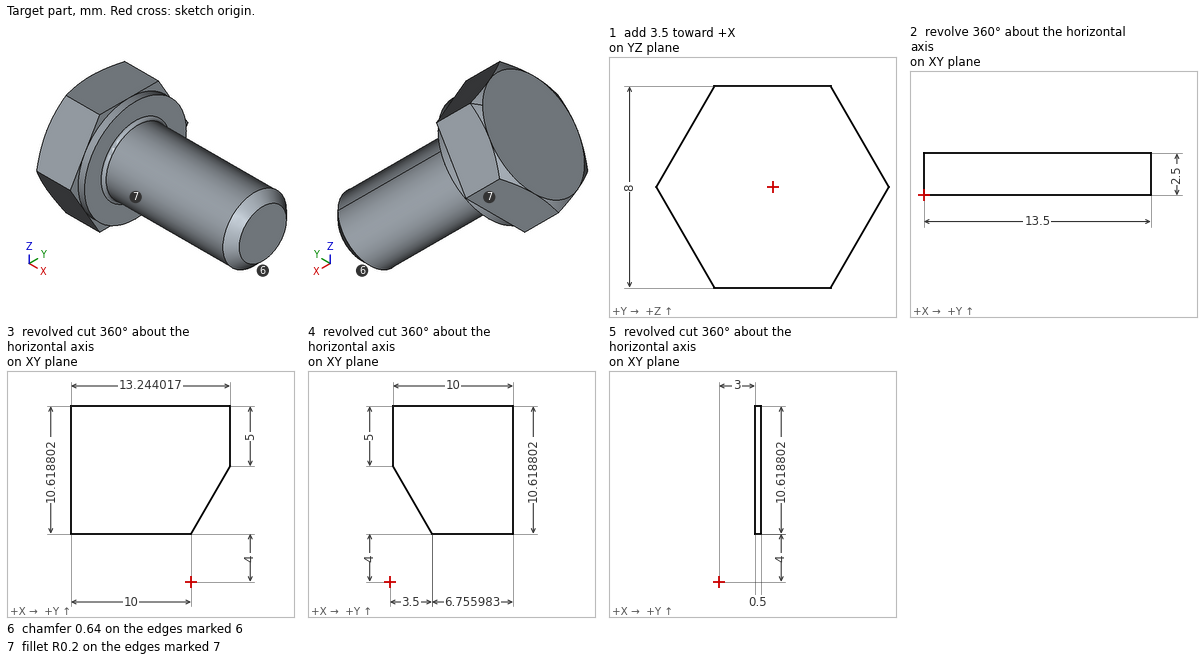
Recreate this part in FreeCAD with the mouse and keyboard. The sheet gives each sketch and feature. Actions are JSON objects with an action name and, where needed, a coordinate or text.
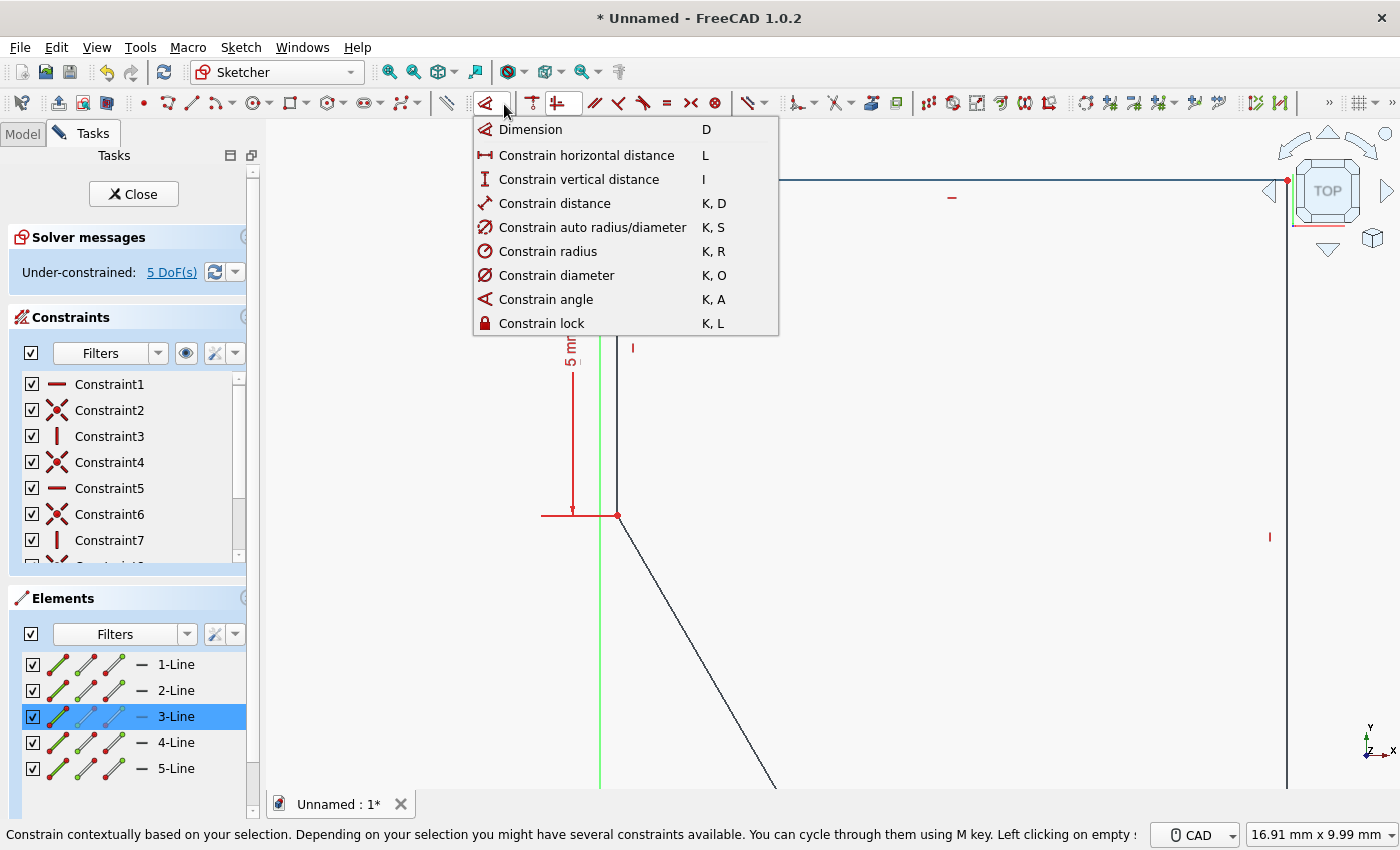
{"action": "left_click", "coordinate": [626, 155]}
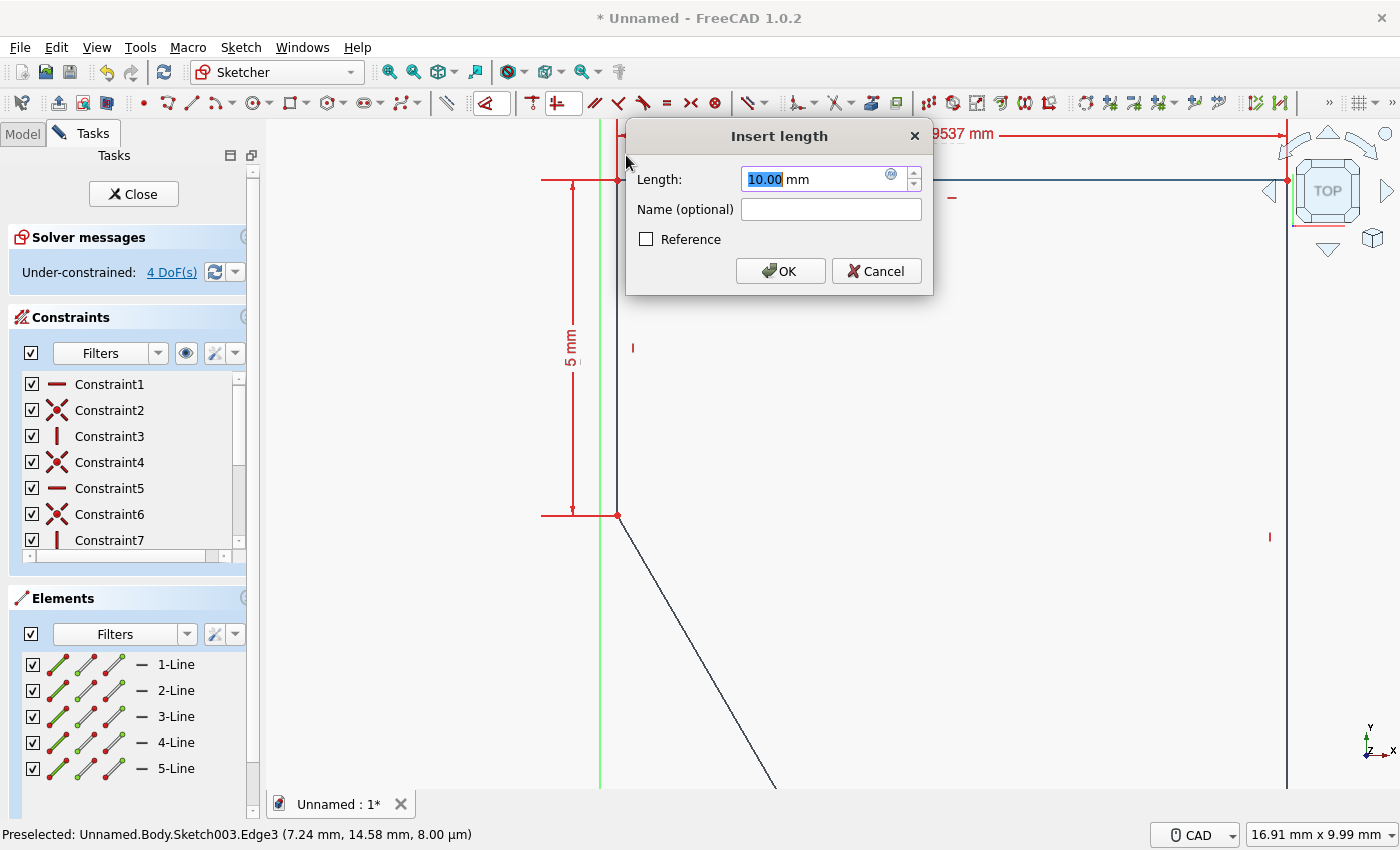
{"action": "type", "text": "10"}
{"action": "key", "text": "Return"}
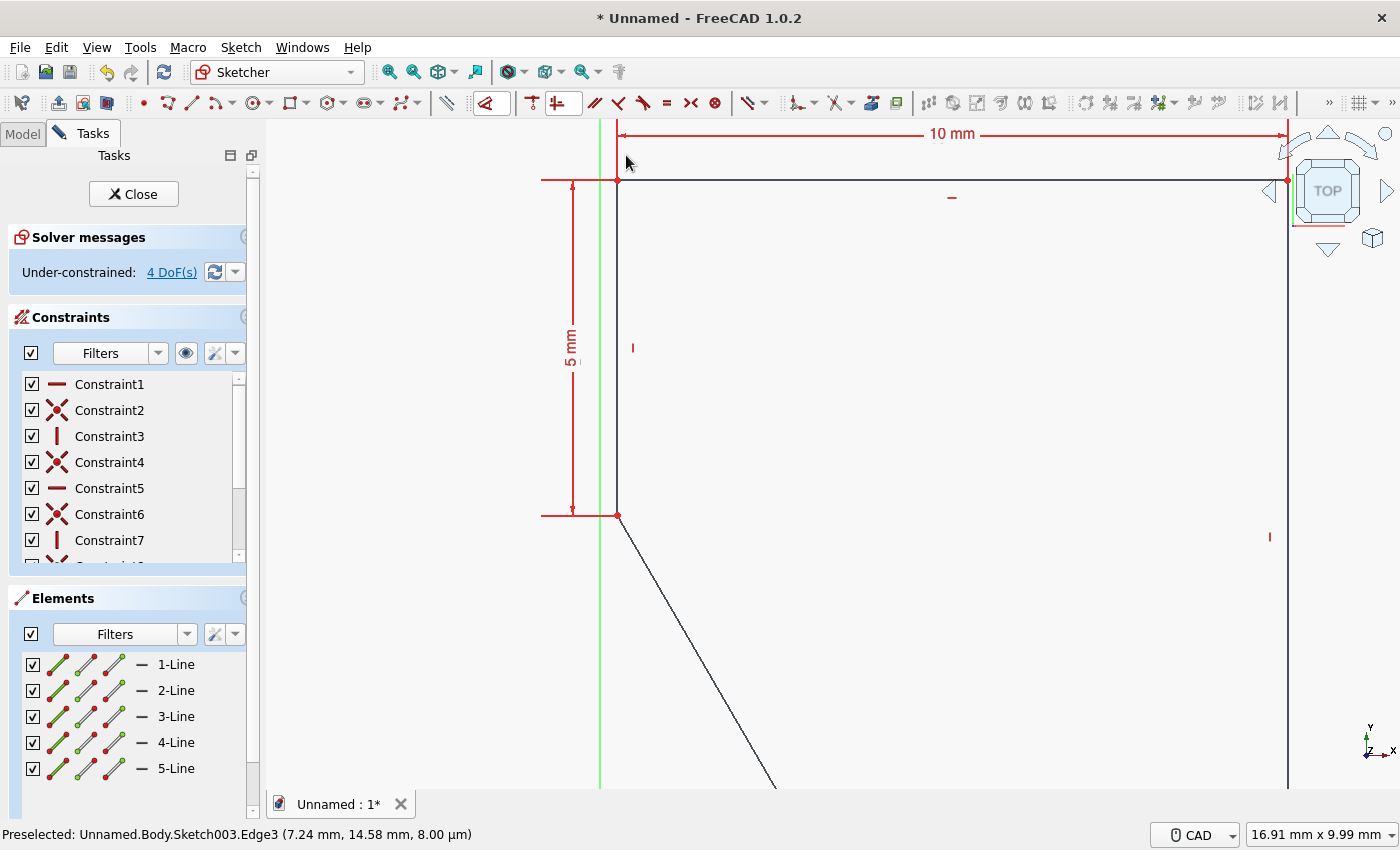
{"action": "scroll", "coordinate": [618, 280], "scroll_direction": "down", "scroll_amount": 4}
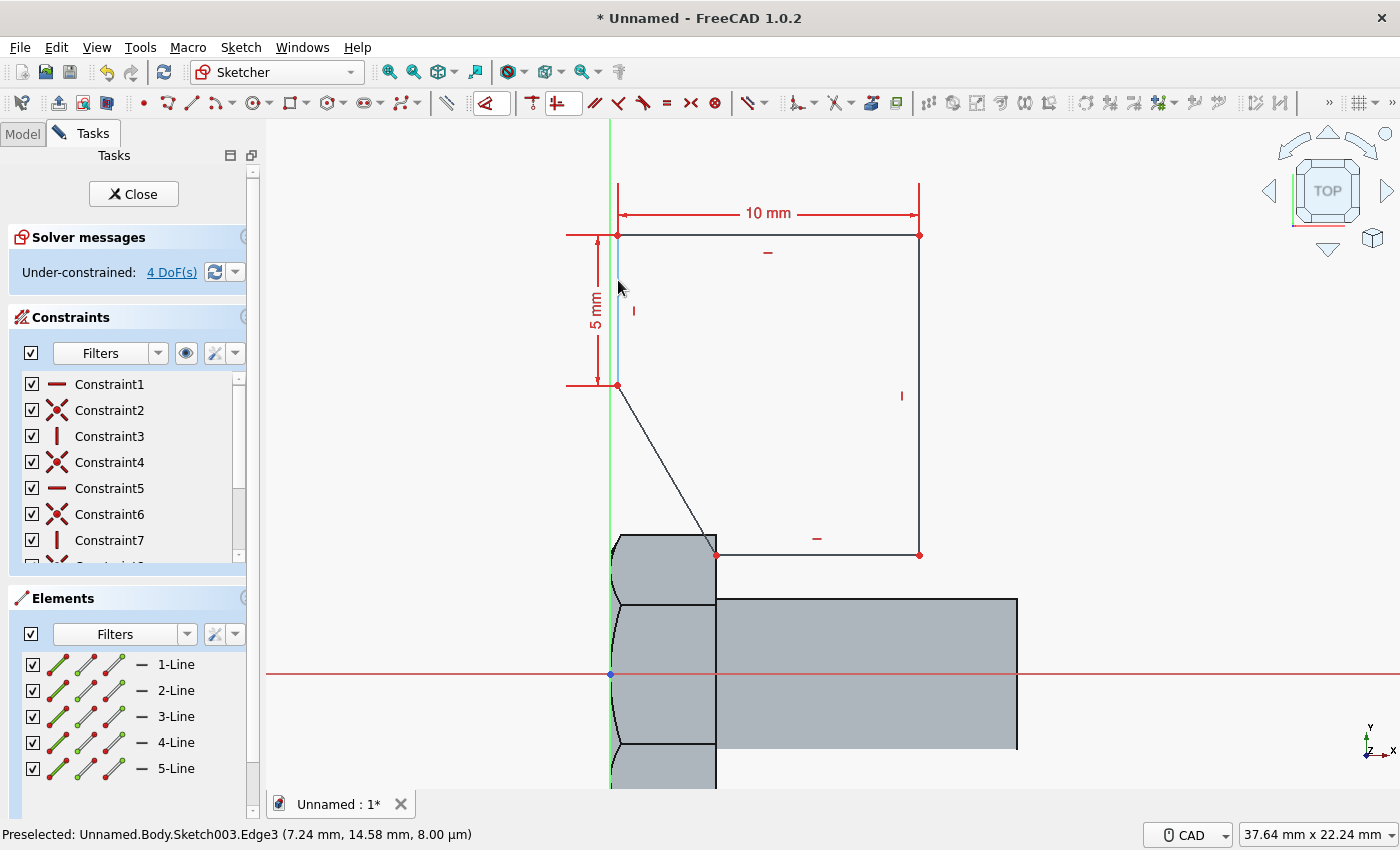
{"action": "left_click", "coordinate": [716, 555]}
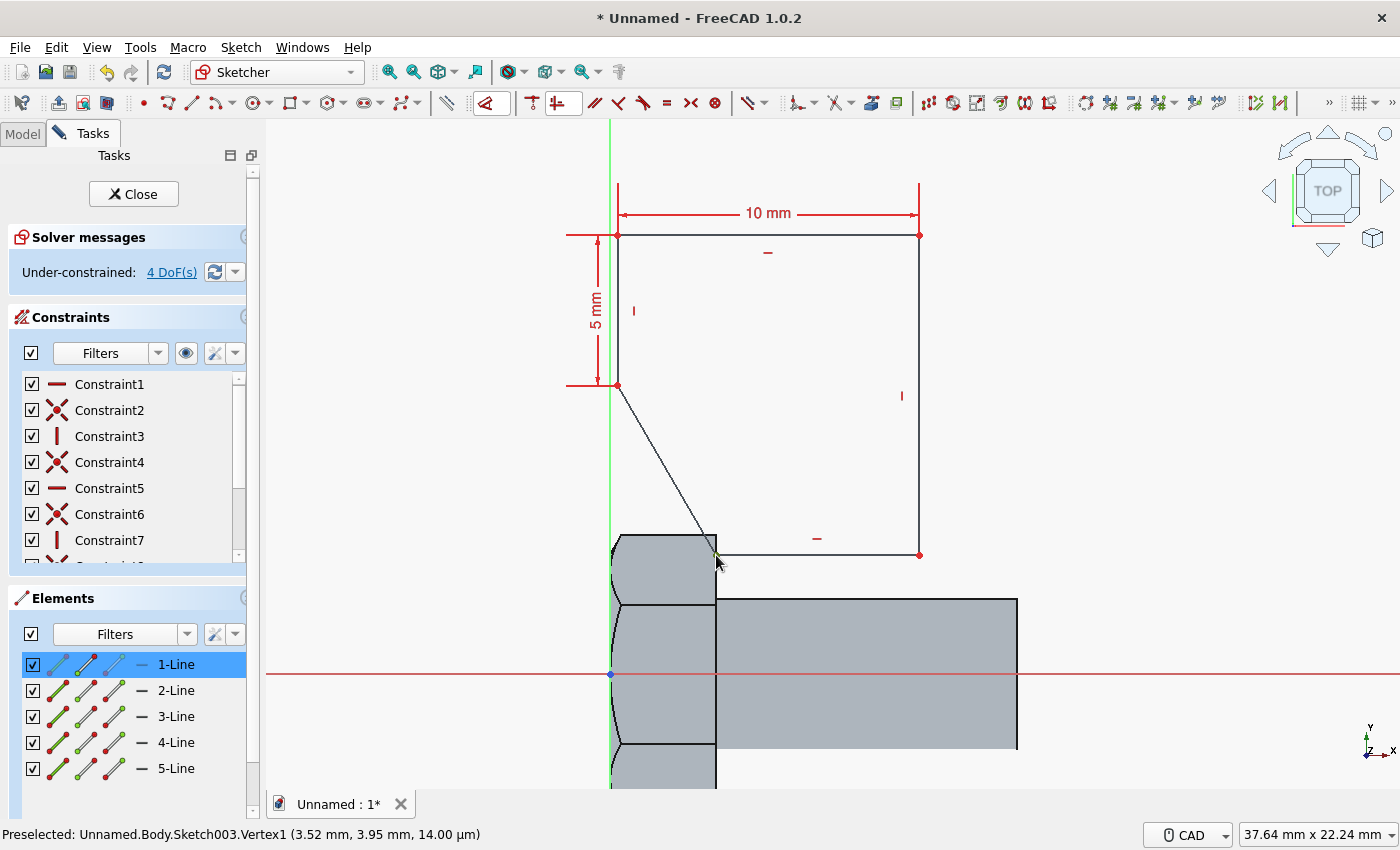
{"action": "key", "text": "i"}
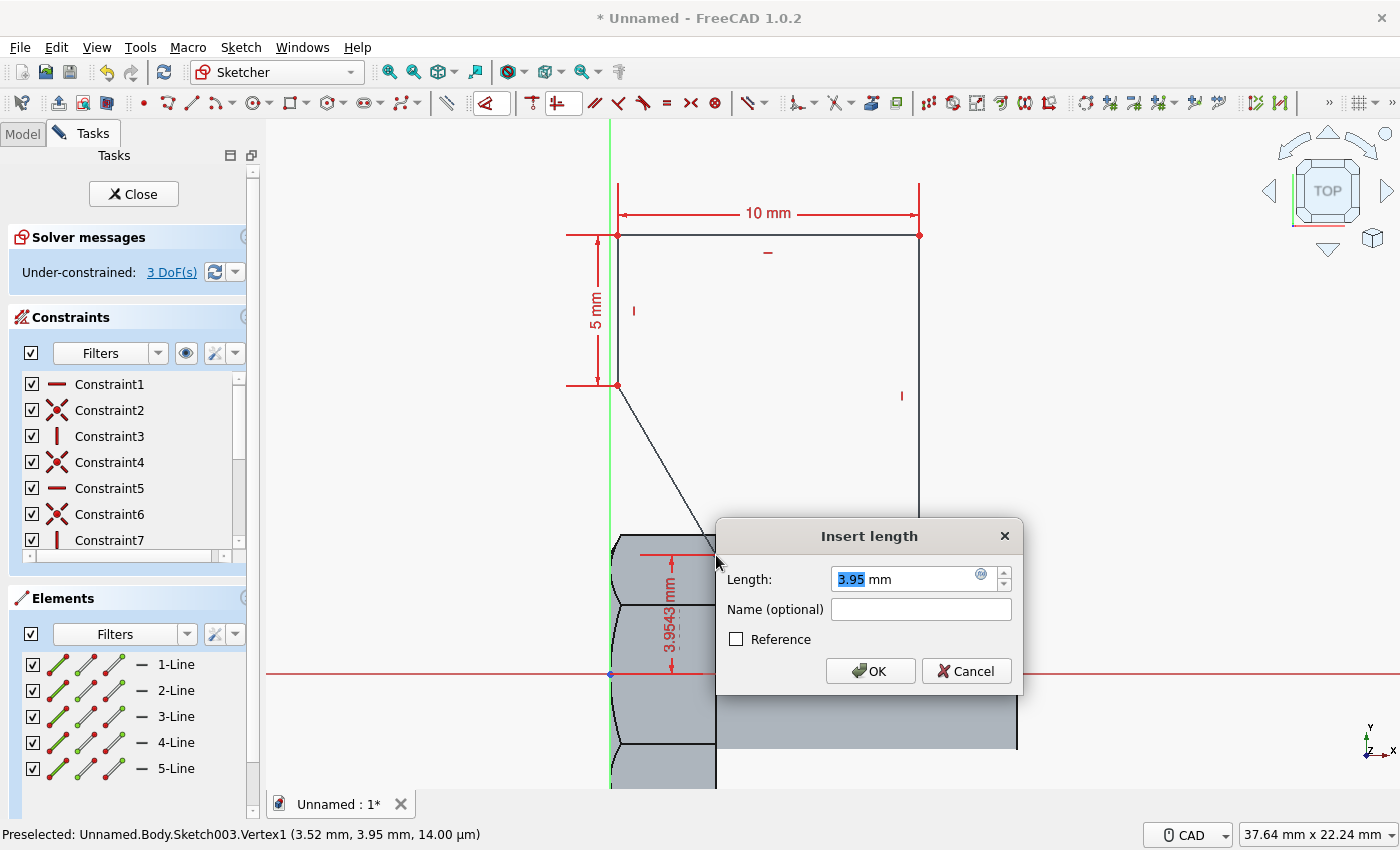
{"action": "type", "text": "4"}
{"action": "key", "text": "Return"}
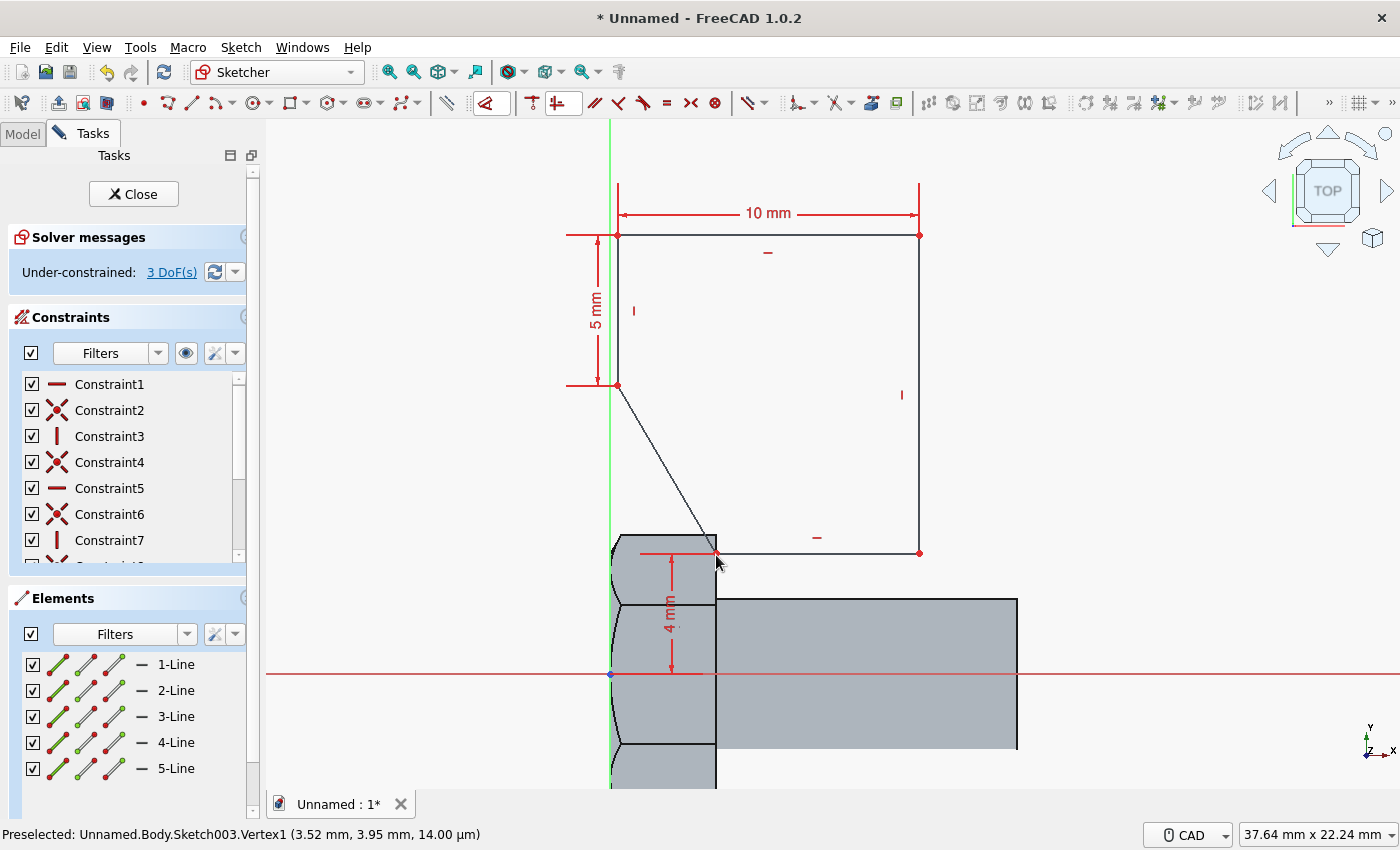
{"action": "left_click", "coordinate": [716, 554]}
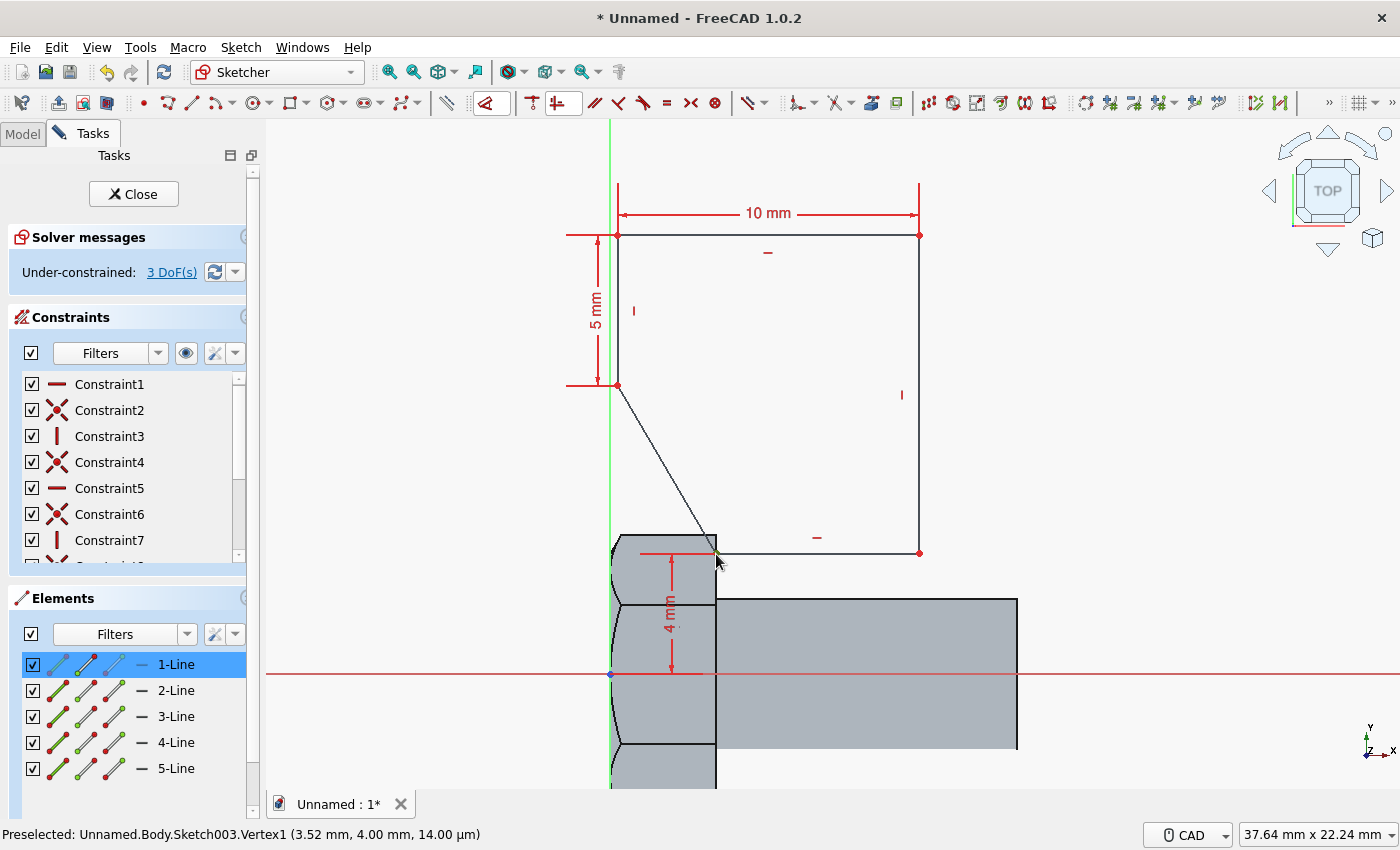
{"action": "left_click", "coordinate": [504, 104]}